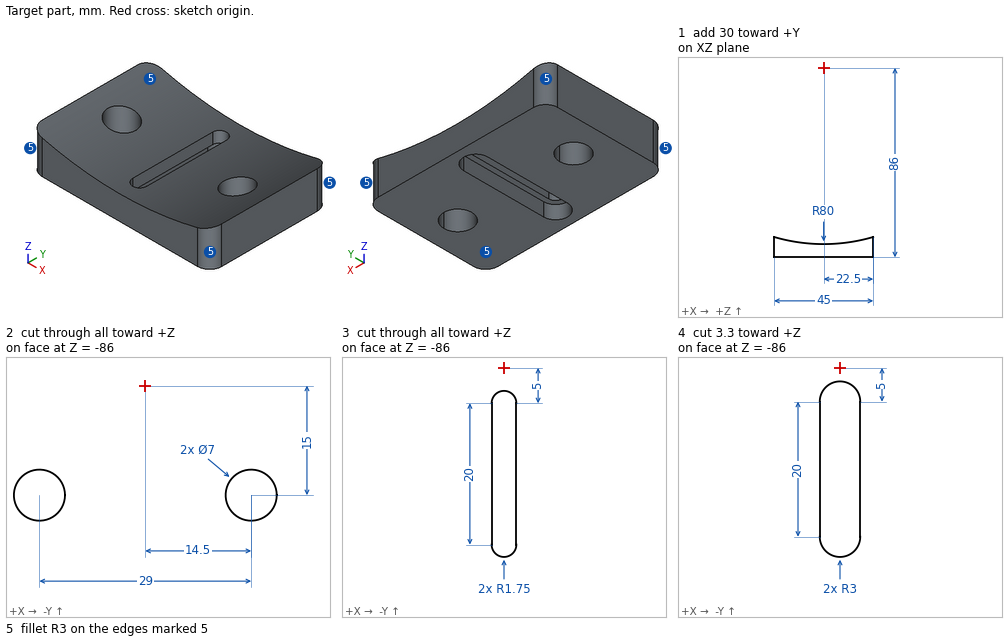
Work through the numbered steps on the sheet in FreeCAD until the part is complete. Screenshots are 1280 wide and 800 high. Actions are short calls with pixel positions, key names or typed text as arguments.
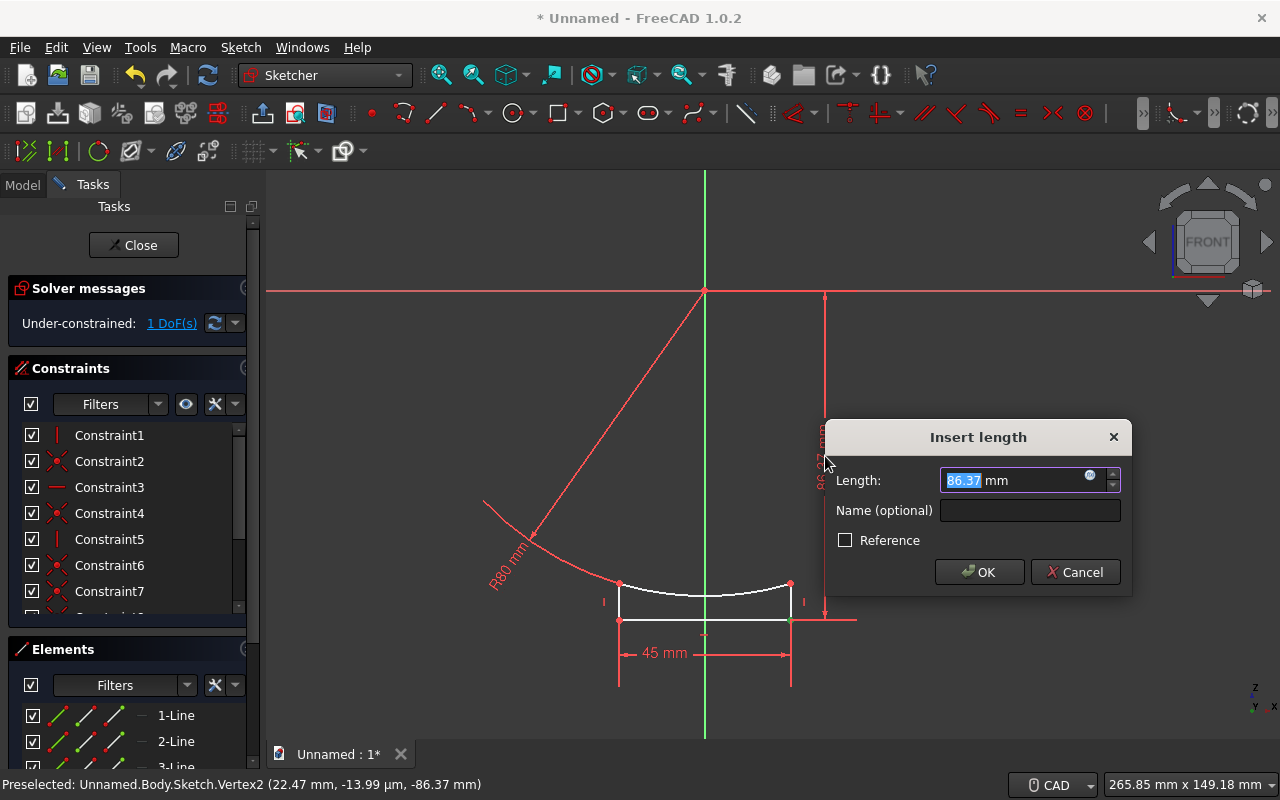
text(86)
key(Return)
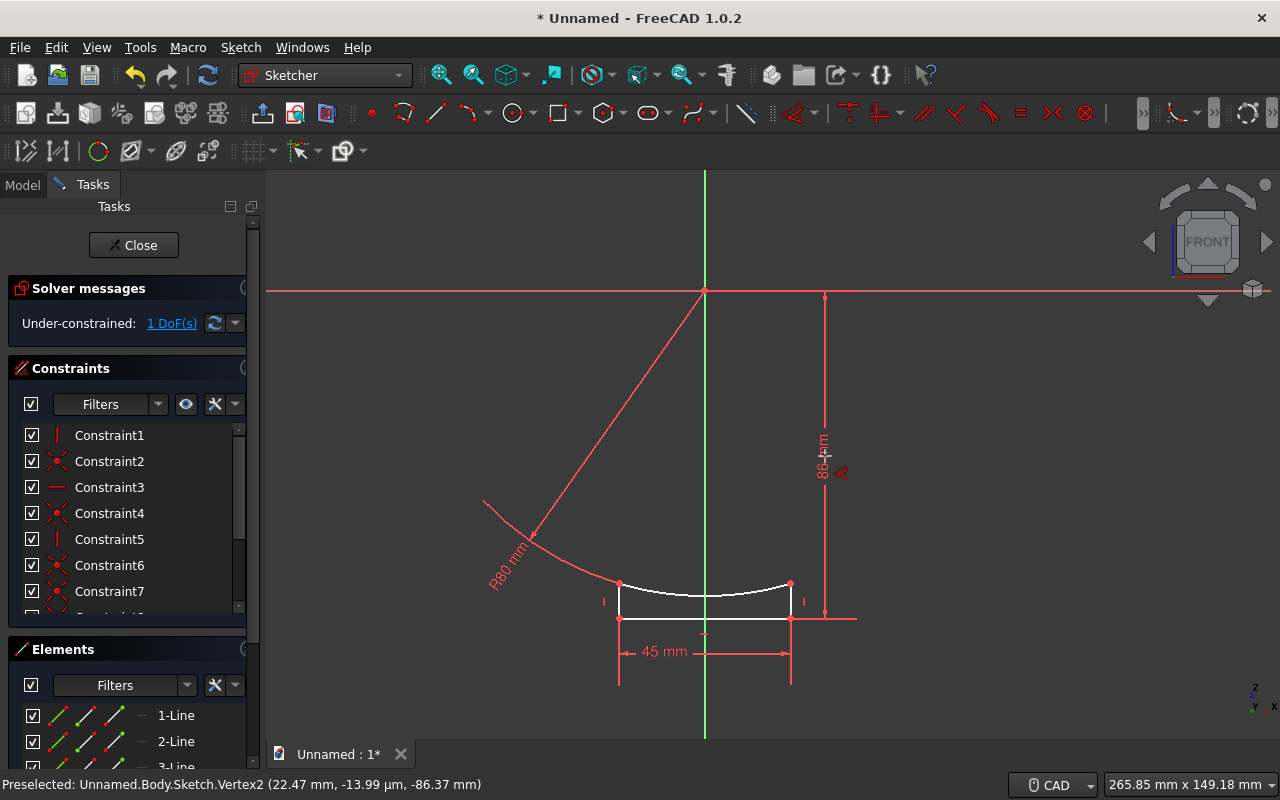
click(791, 584)
click(748, 257)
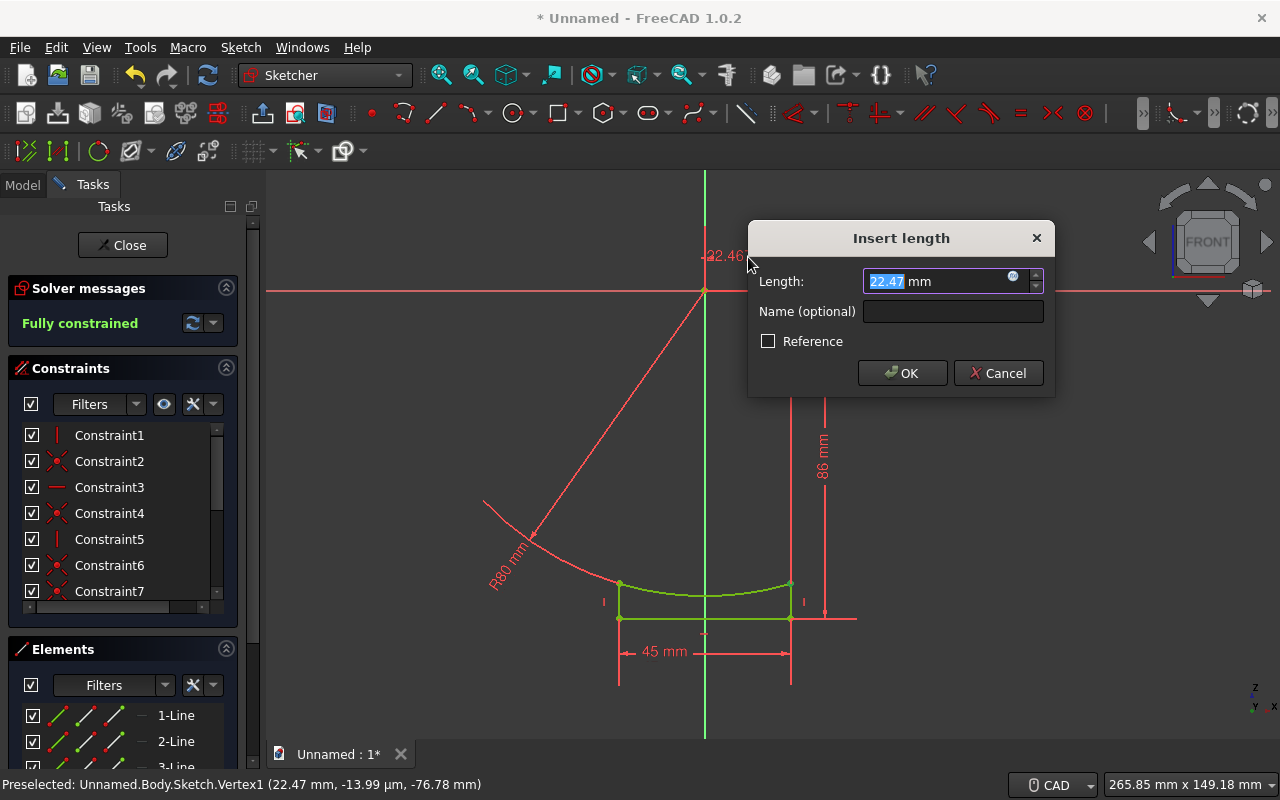
text(22.5)
key(Return)
key(Escape)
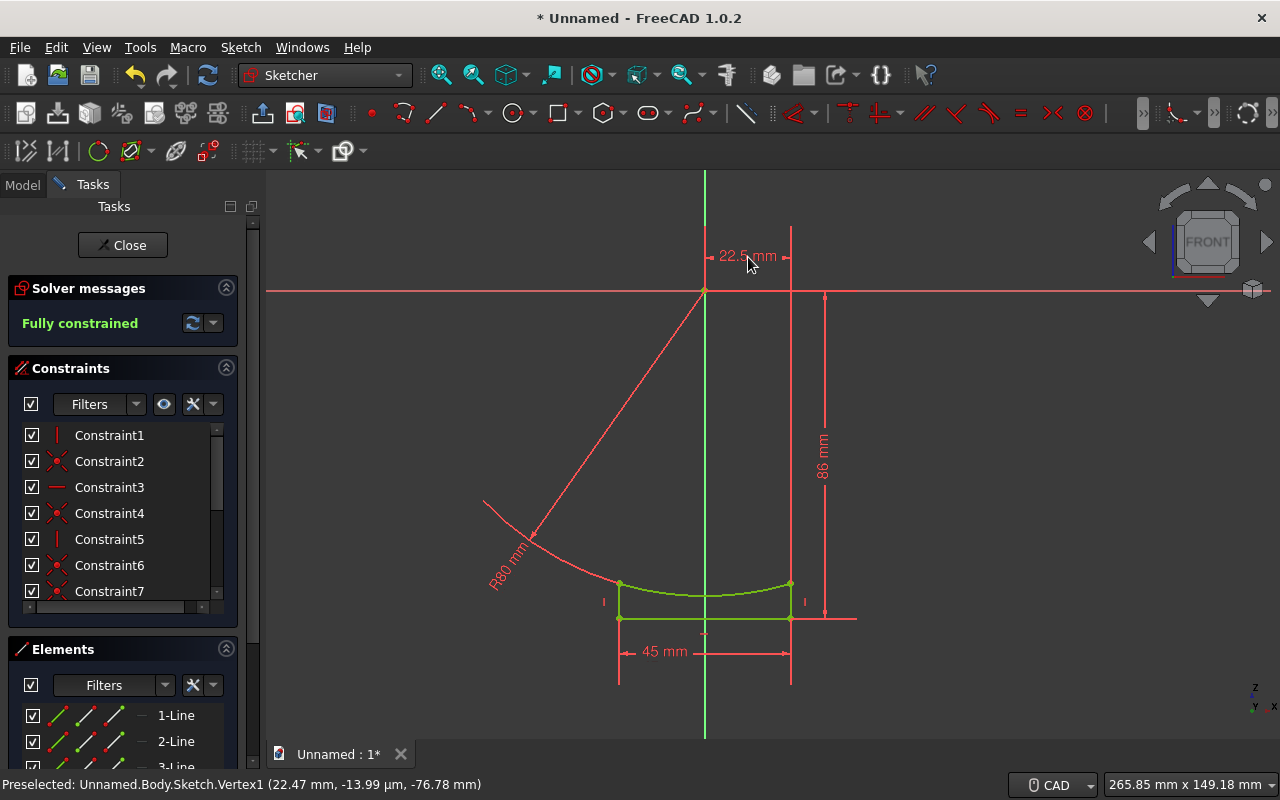
click(123, 245)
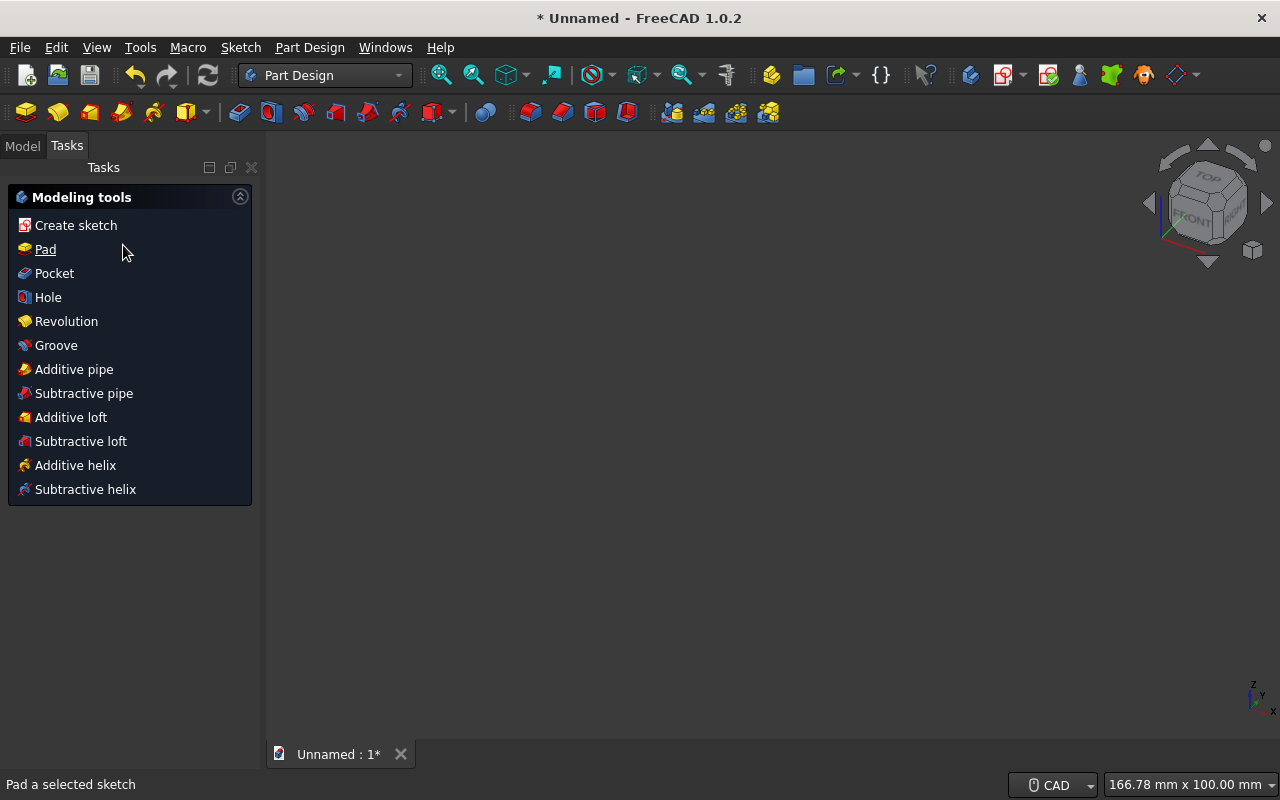
click(26, 112)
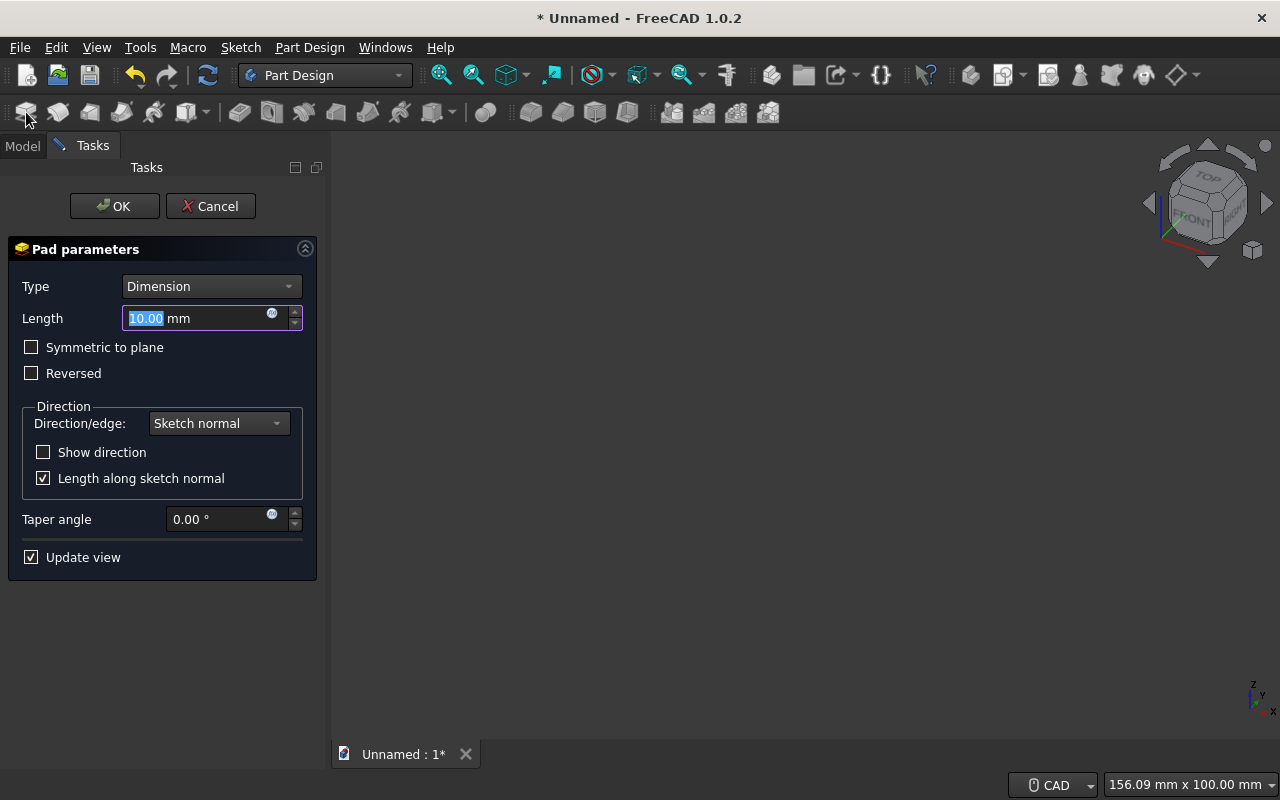
text(30)
key(Tab)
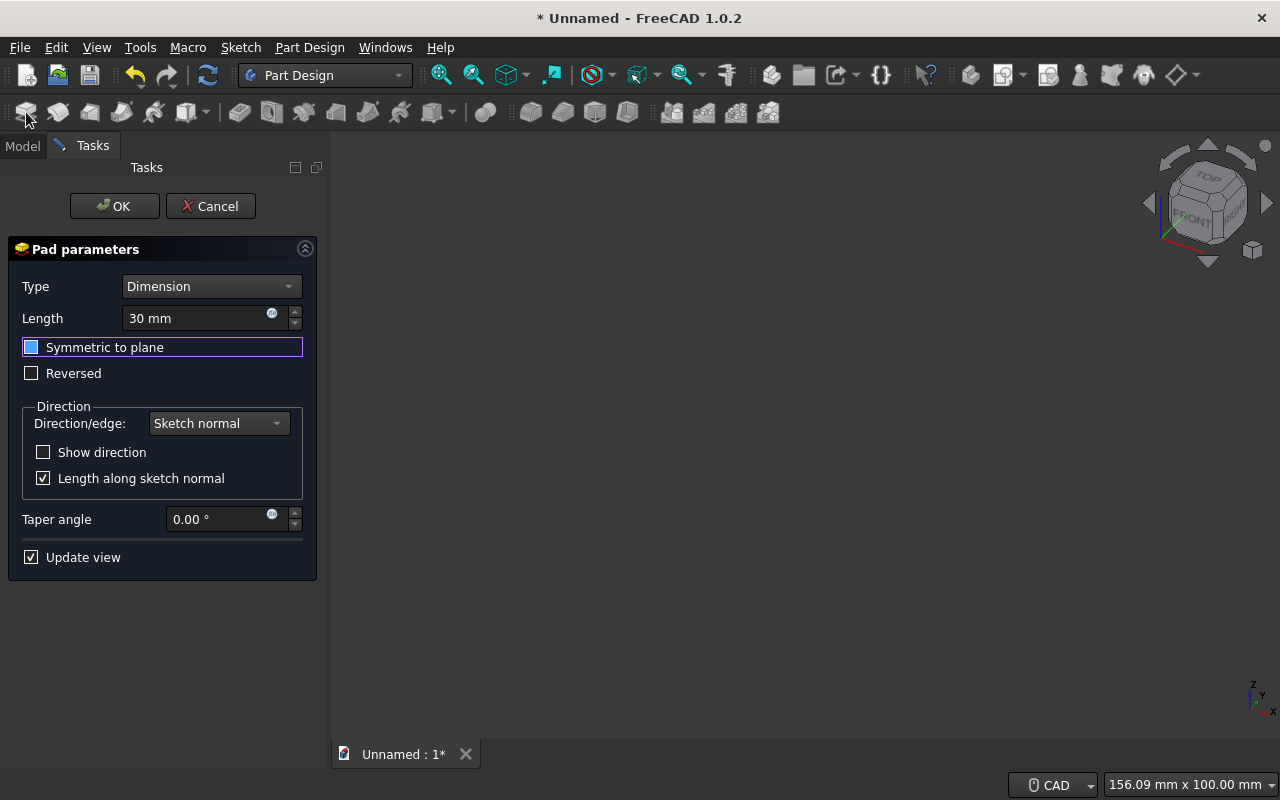
click(30, 373)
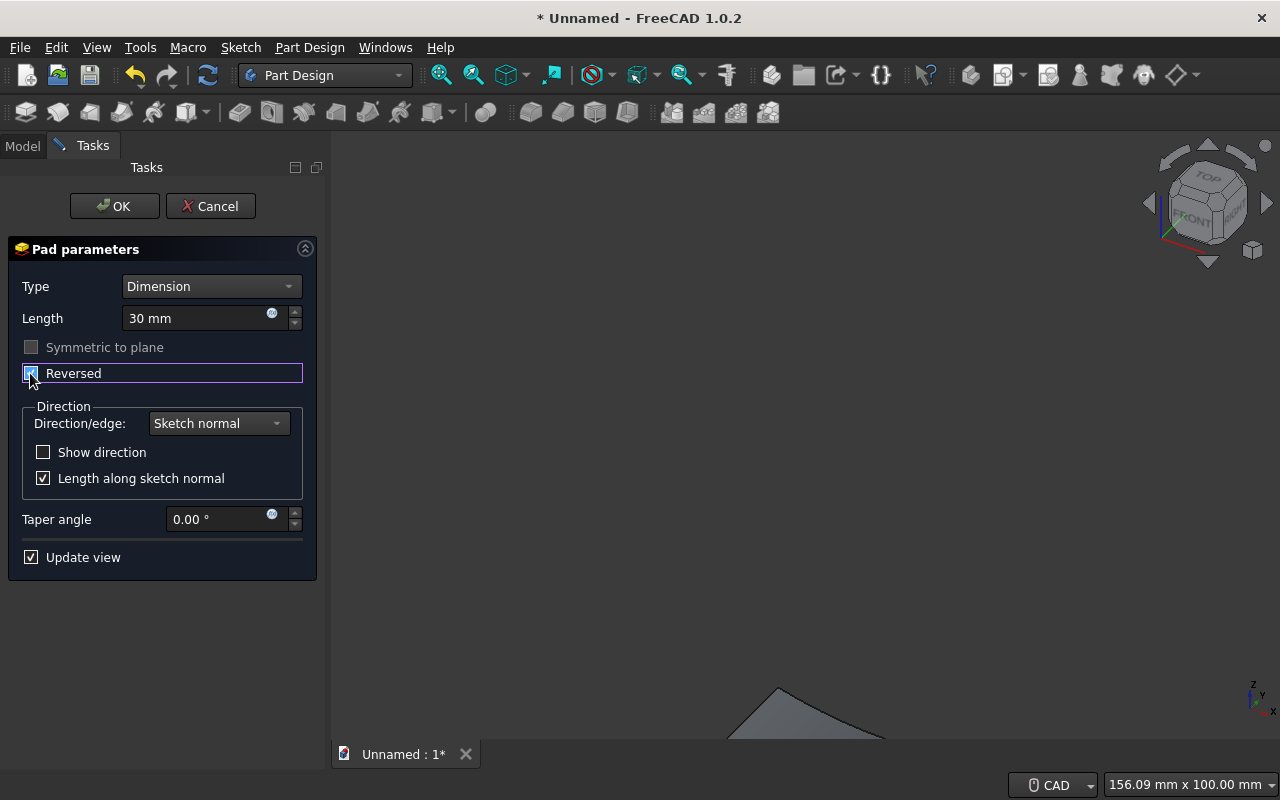
click(115, 206)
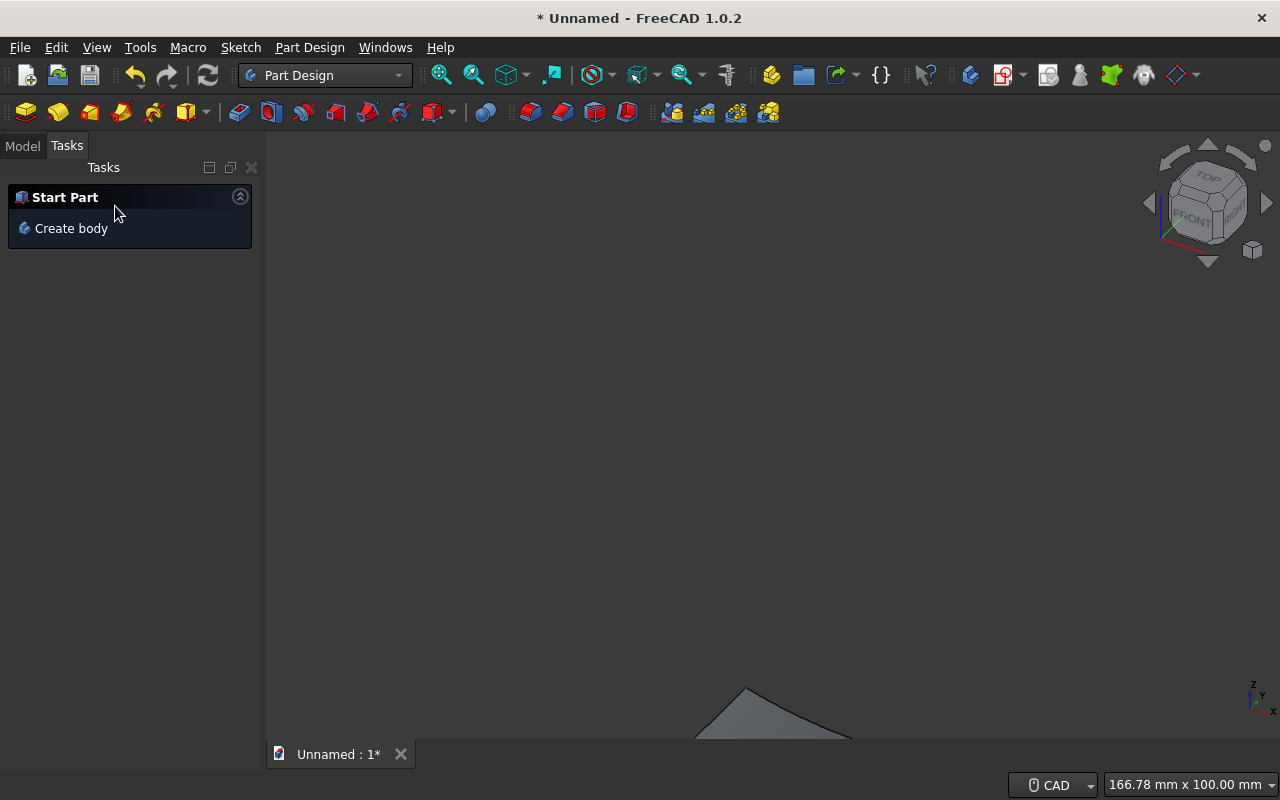
click(442, 76)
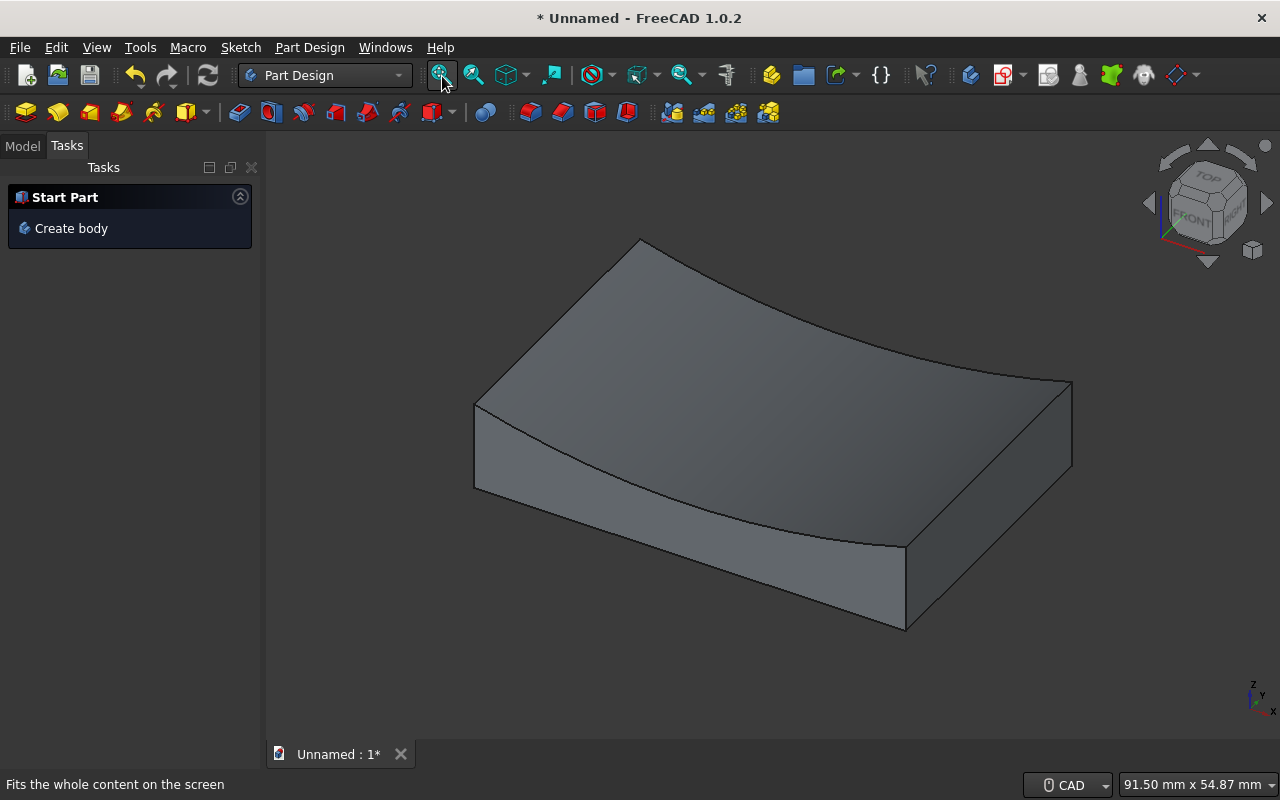
key(5)